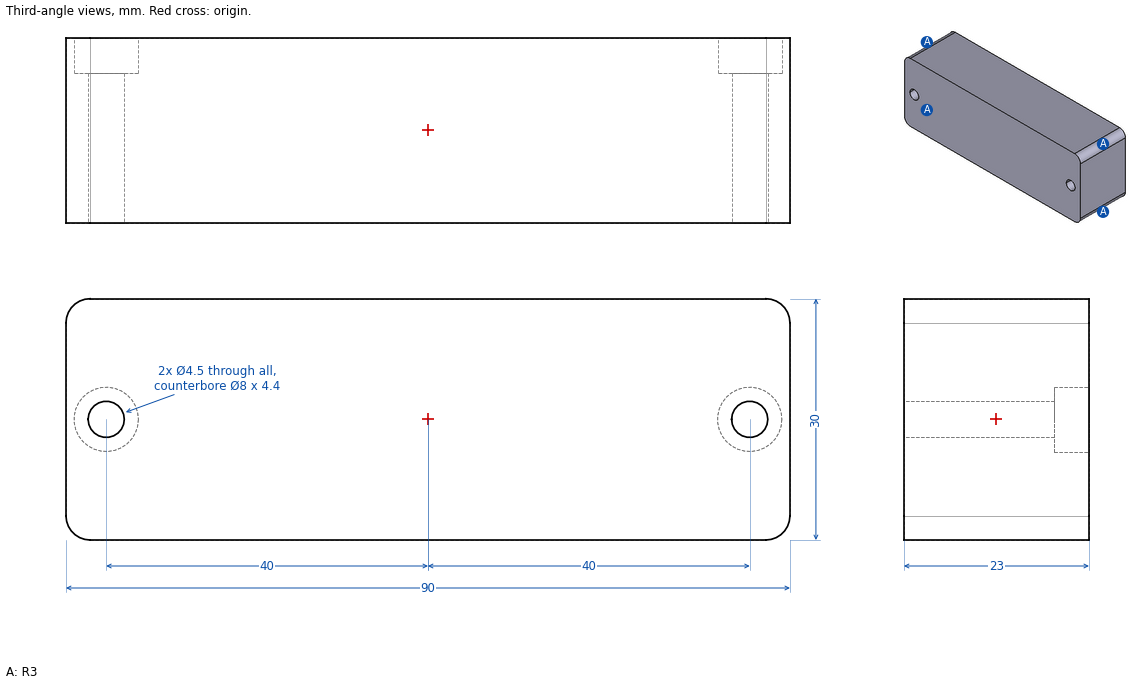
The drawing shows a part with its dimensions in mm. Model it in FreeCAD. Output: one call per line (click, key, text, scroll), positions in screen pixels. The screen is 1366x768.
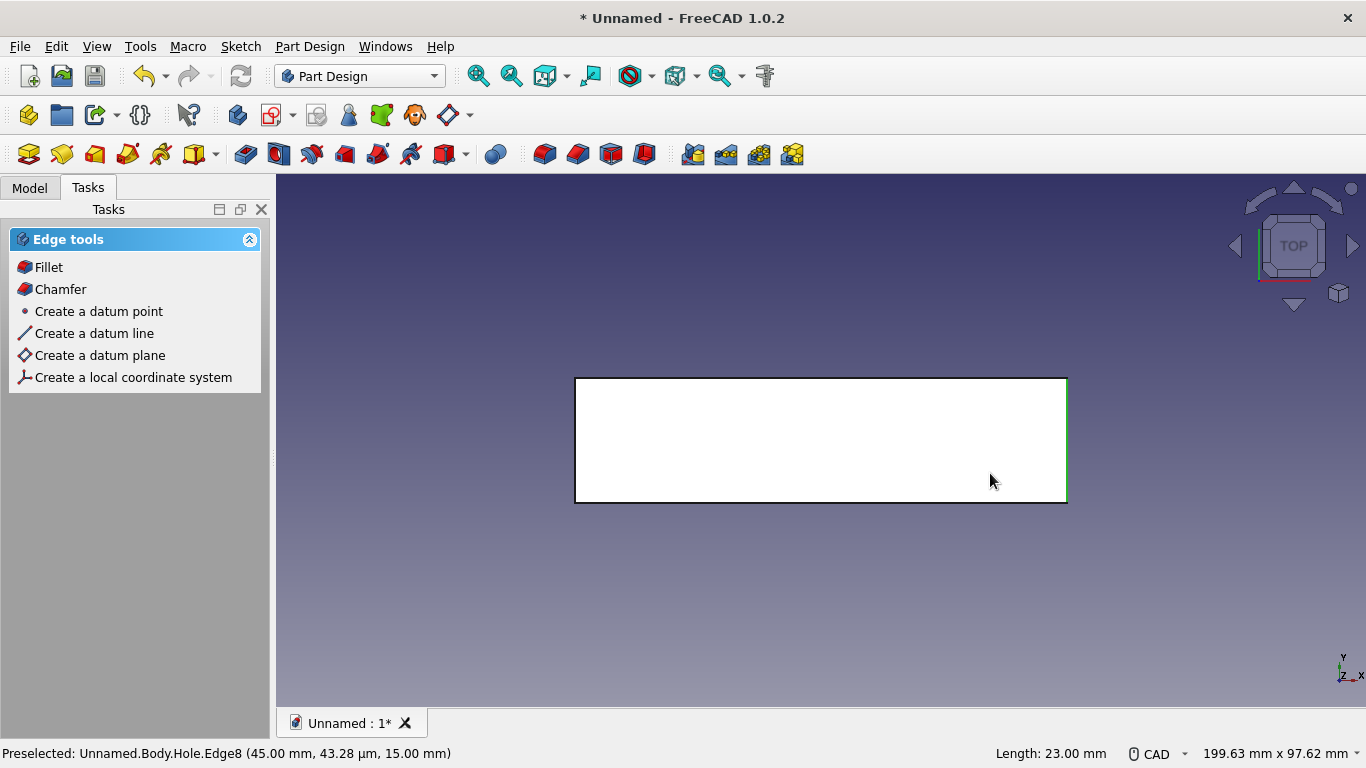
click(575, 439, ctrl)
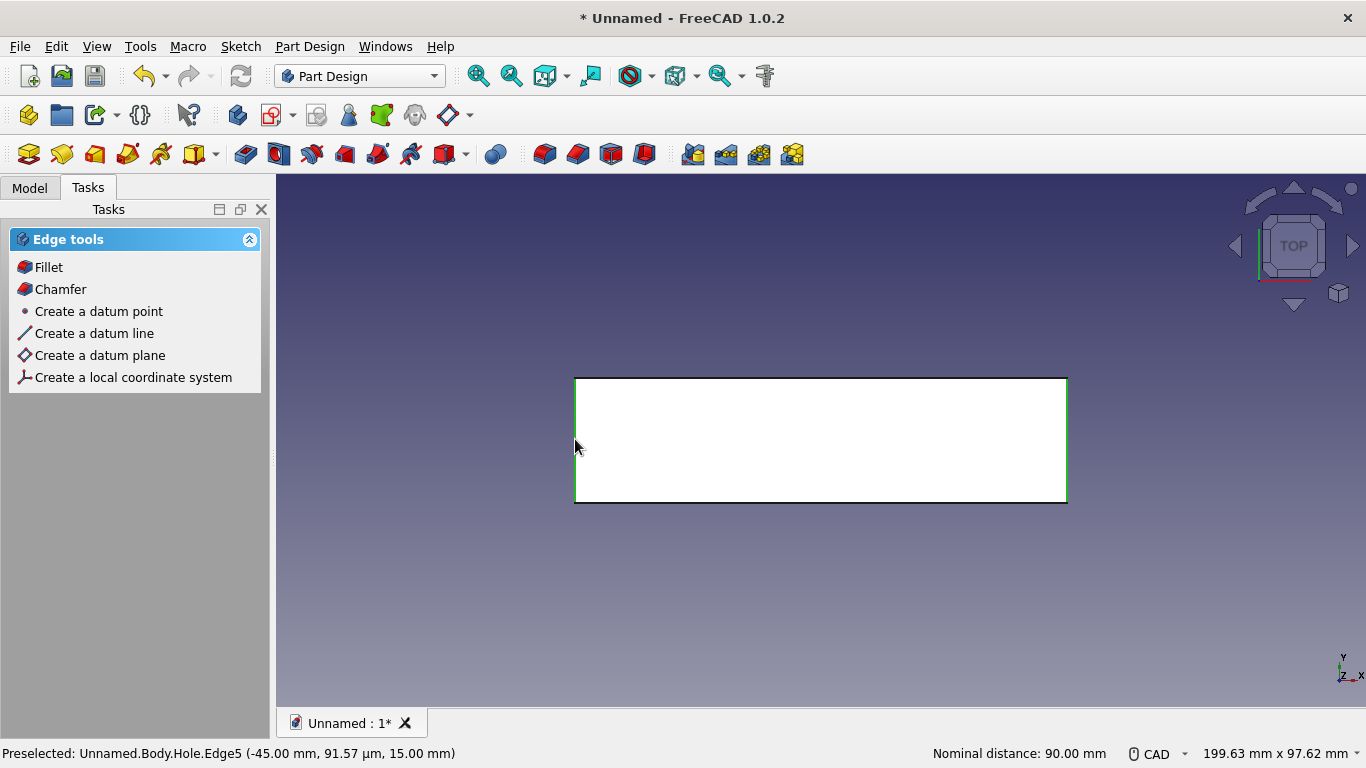
key(1)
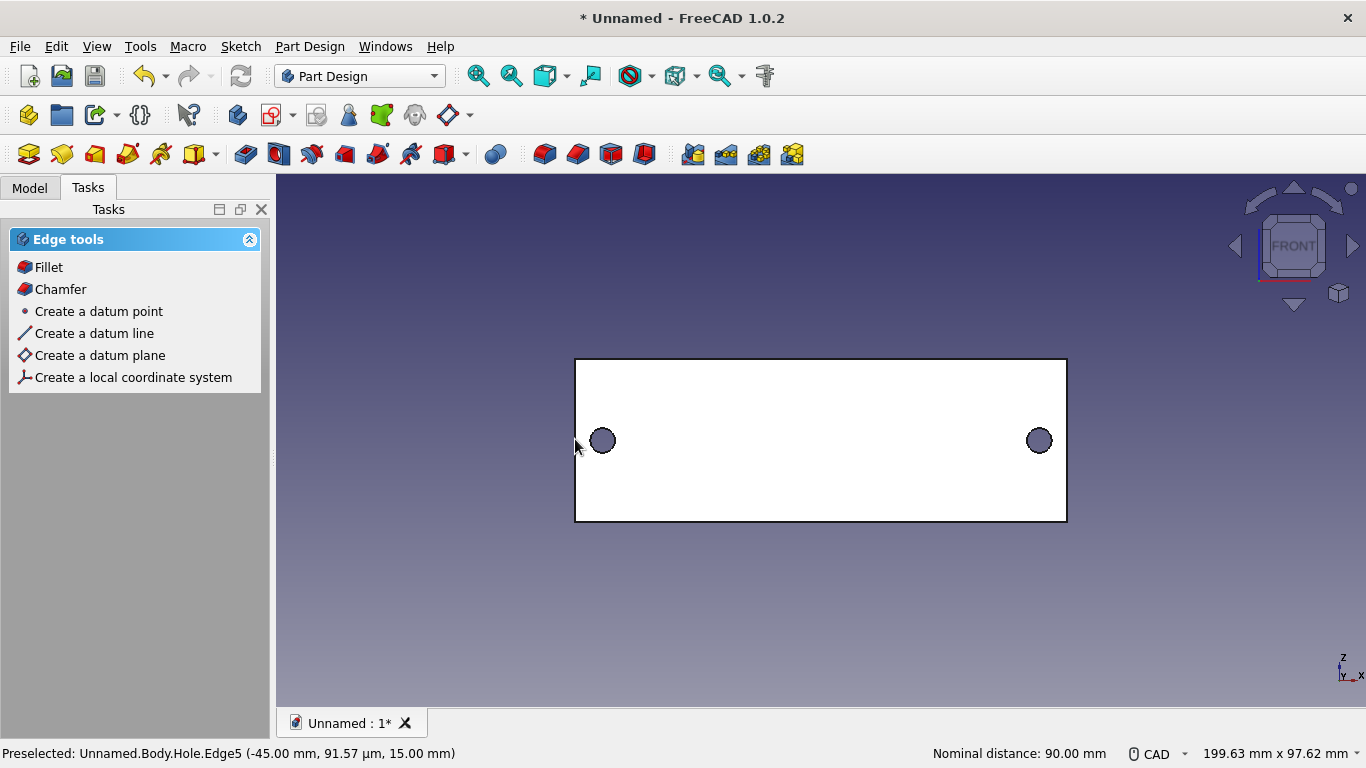
key(3)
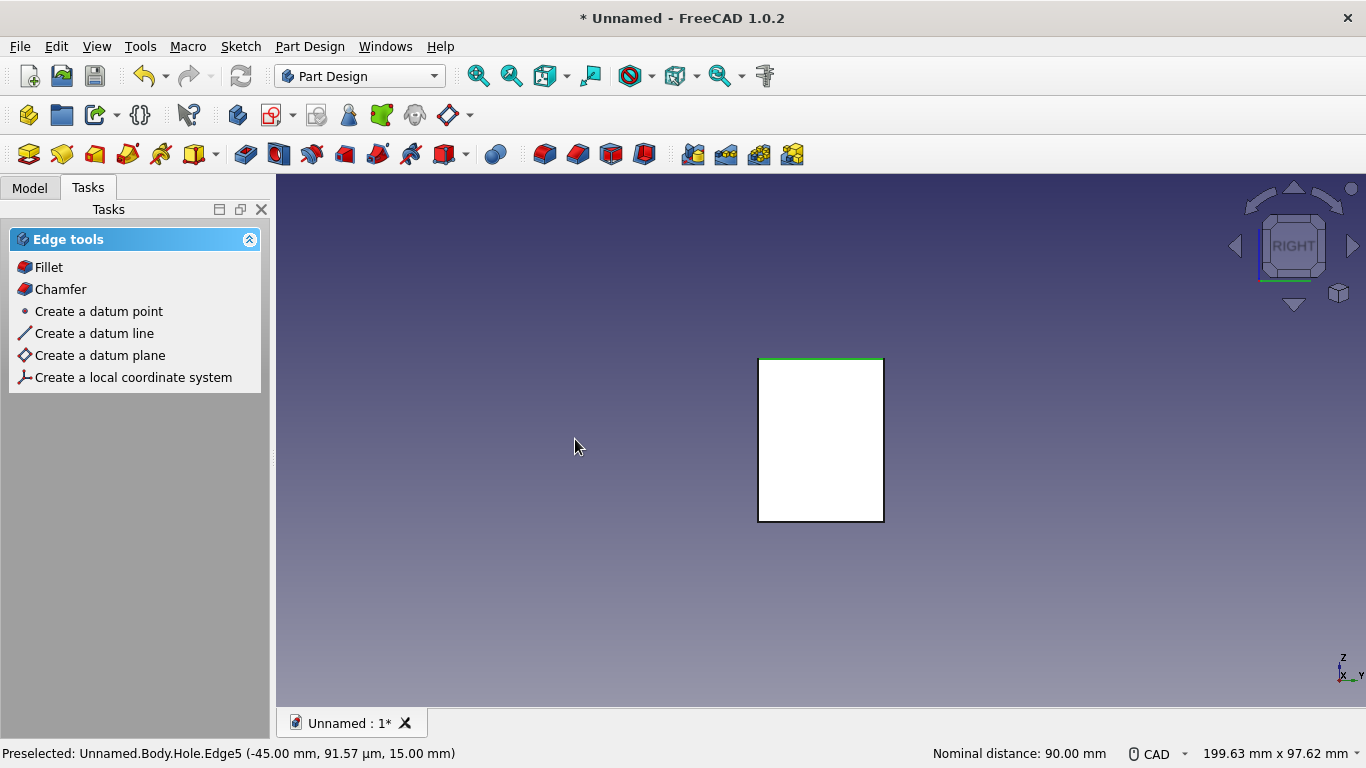
key(v)
key(f)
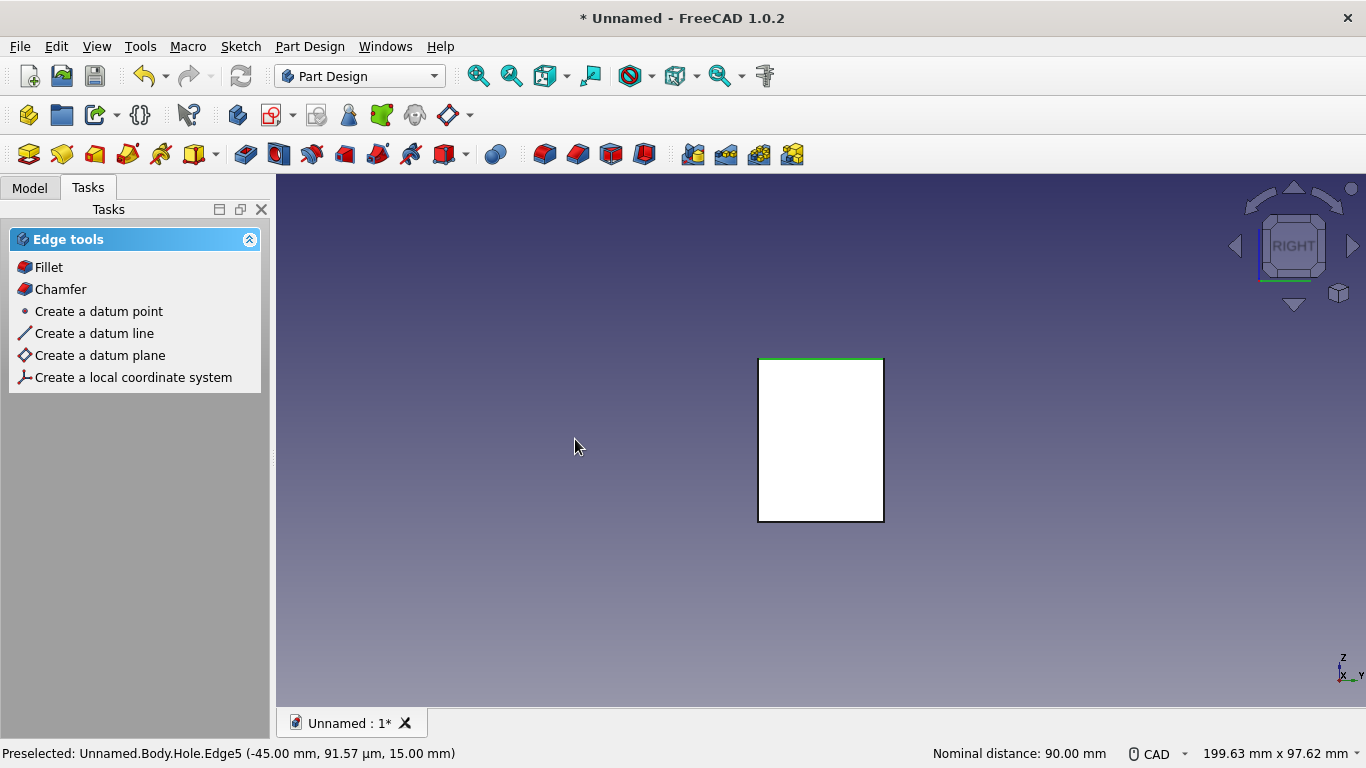
click(821, 521, ctrl)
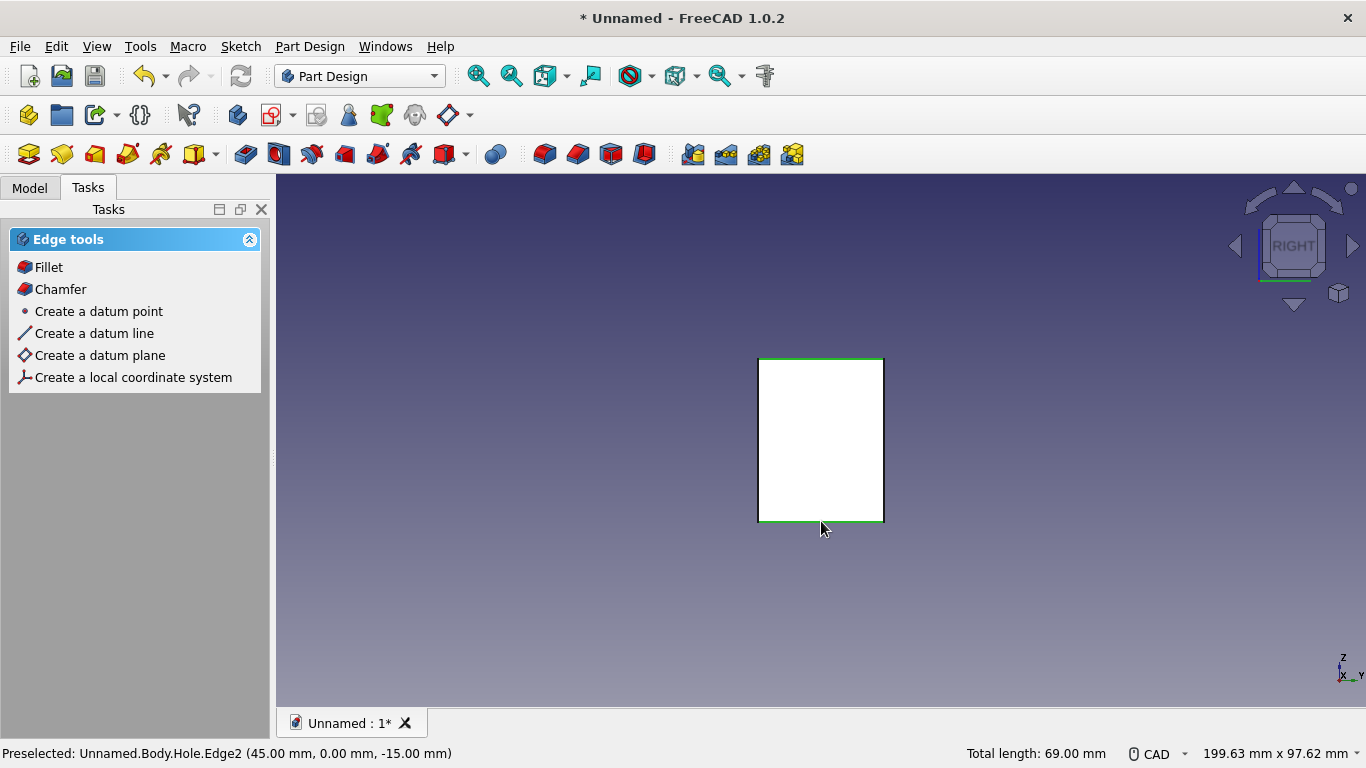
key(5)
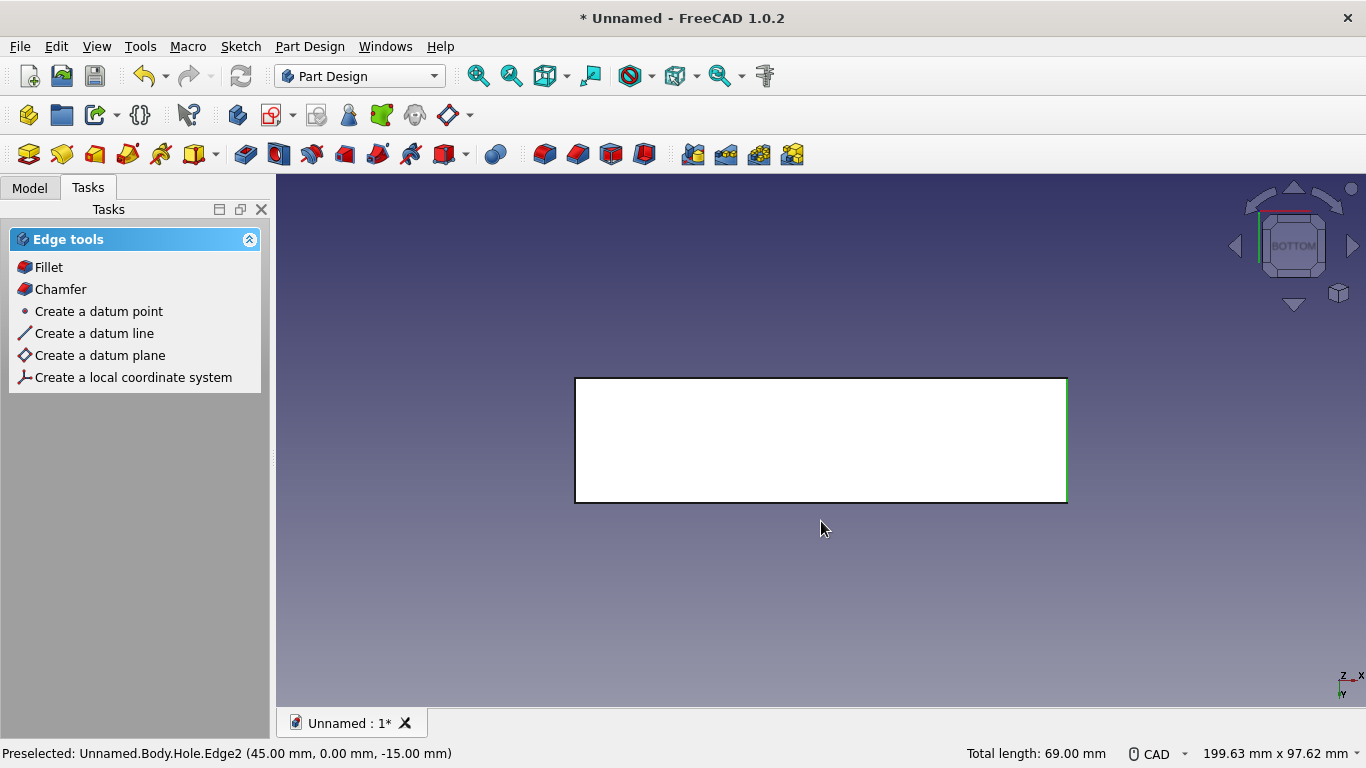
click(575, 439, ctrl)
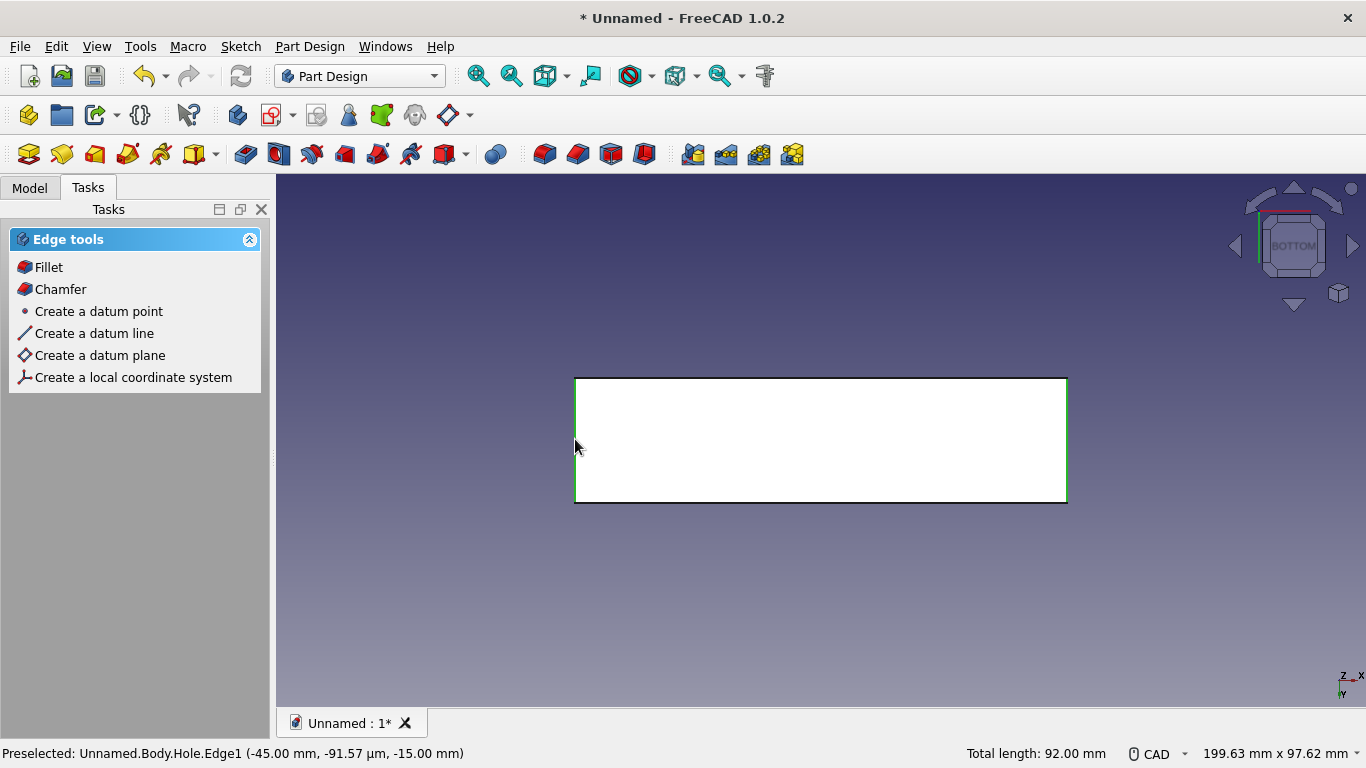
click(545, 154)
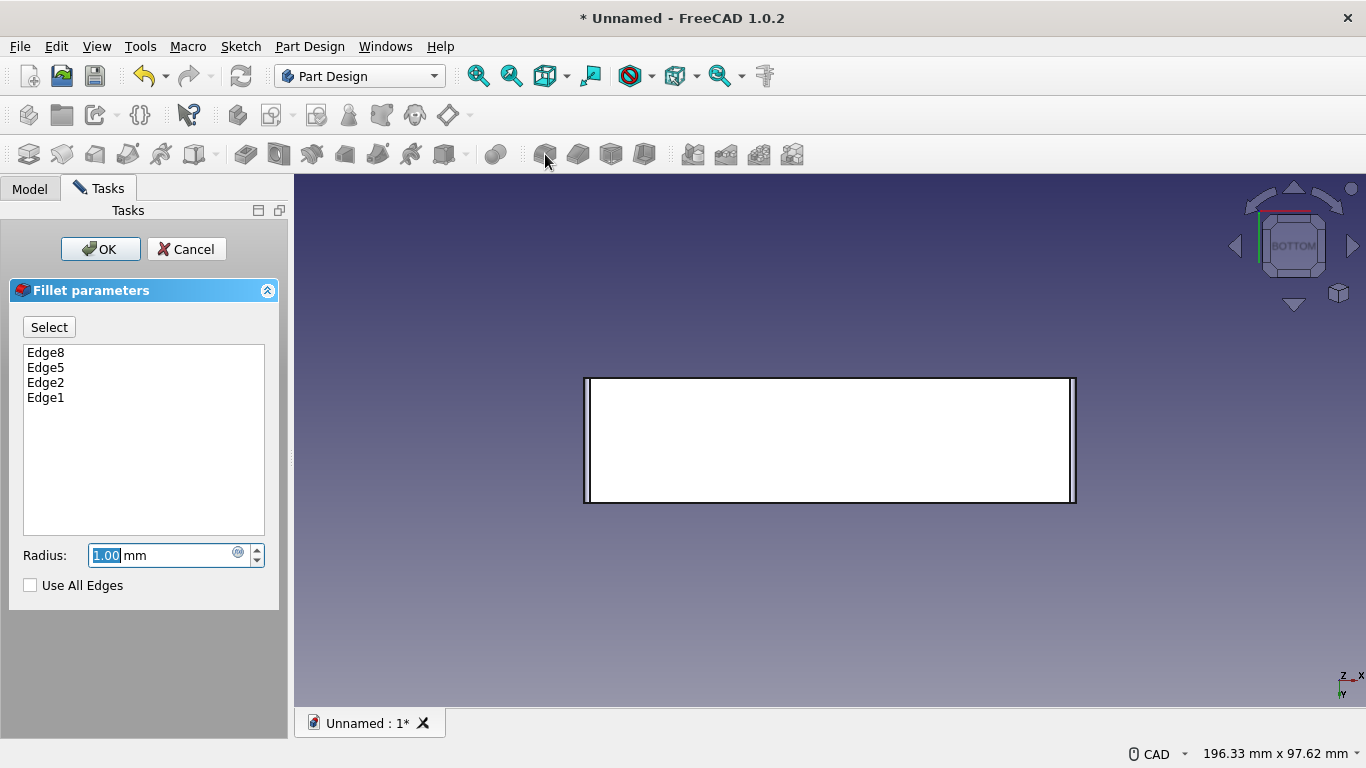
text(3)
key(Tab)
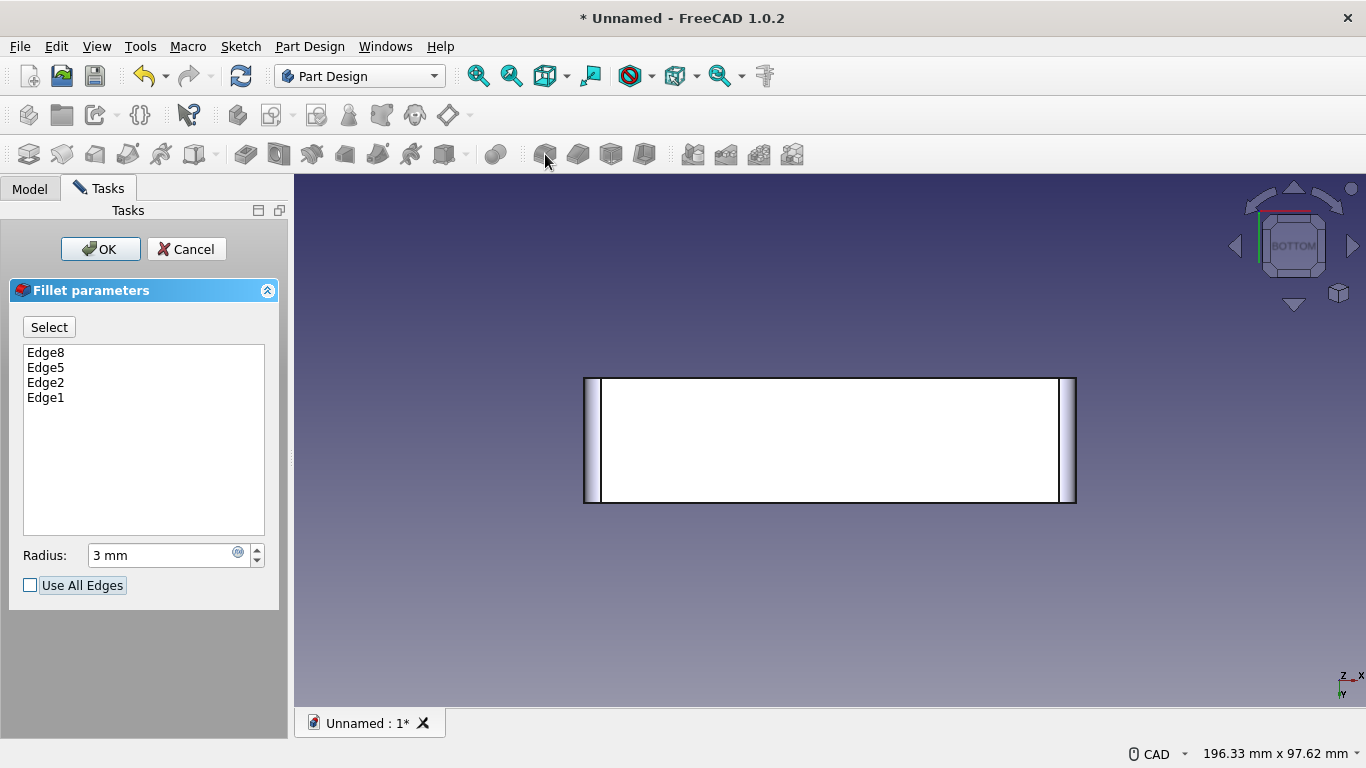
click(101, 249)